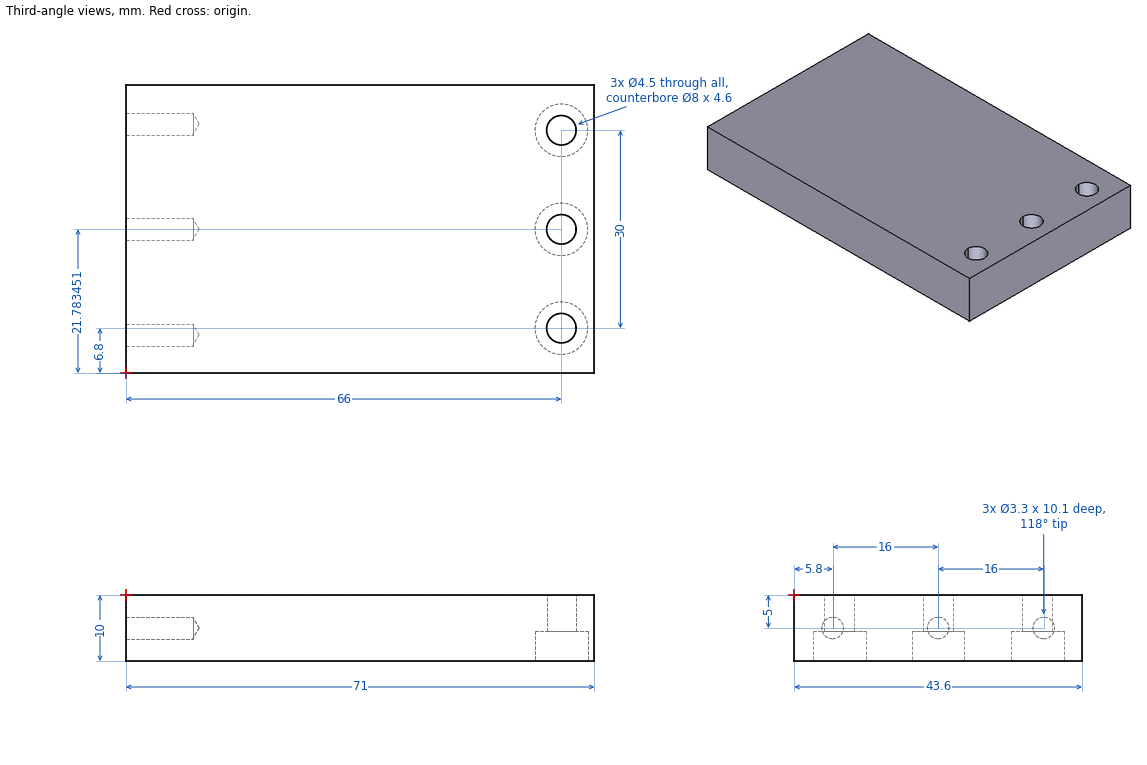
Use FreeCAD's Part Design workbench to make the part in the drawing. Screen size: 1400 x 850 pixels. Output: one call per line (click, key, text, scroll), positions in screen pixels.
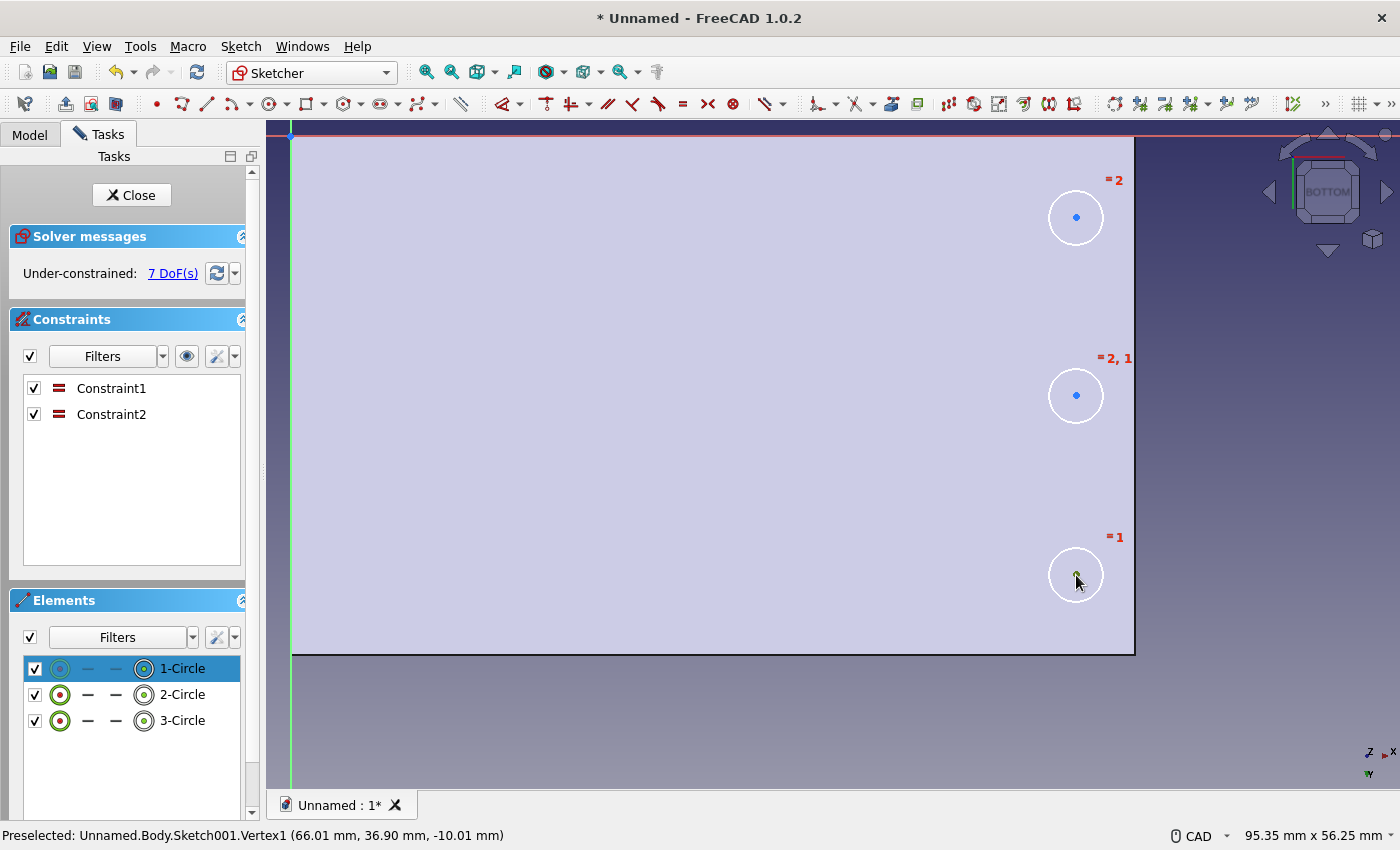
click(1076, 396)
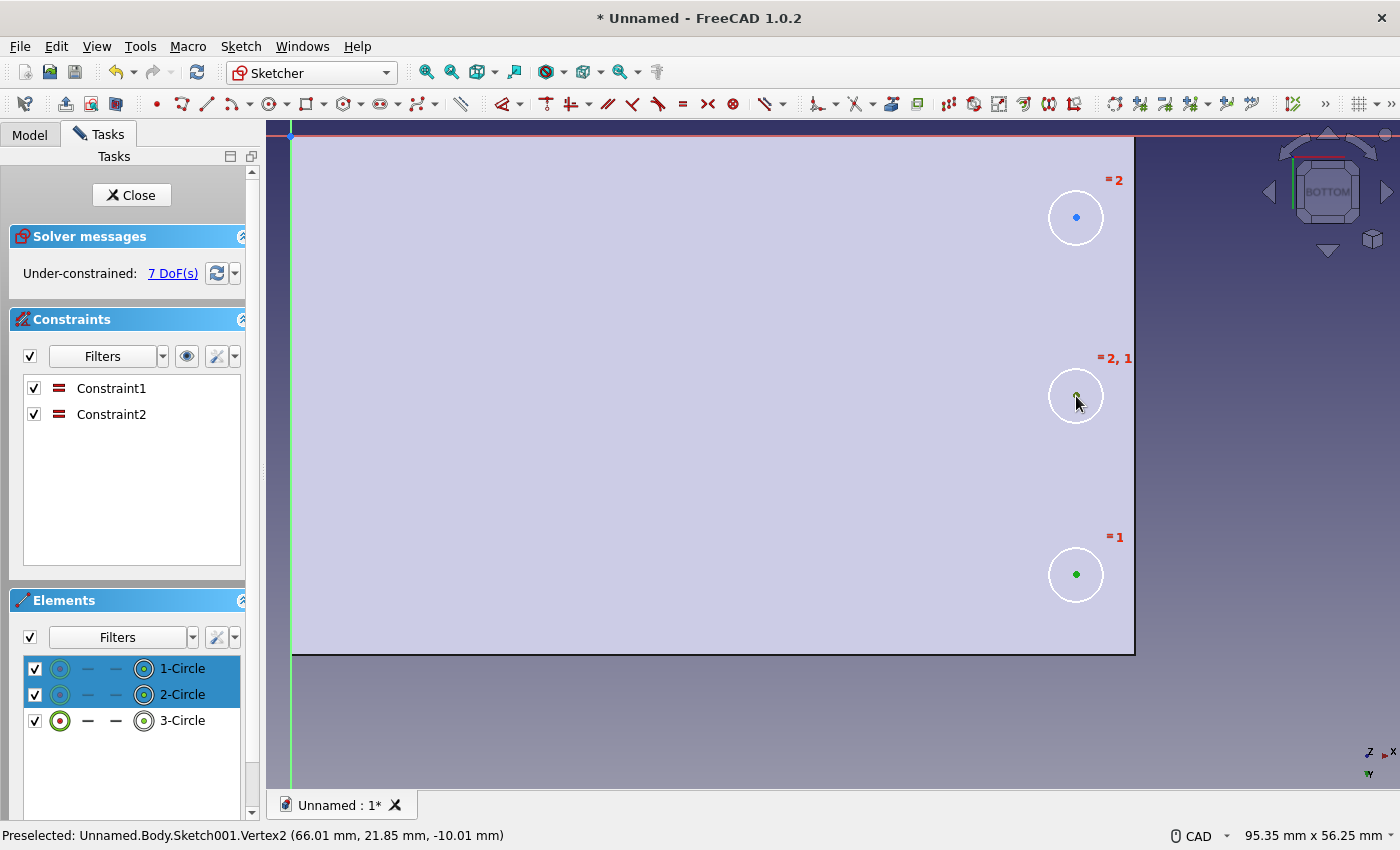
key(v)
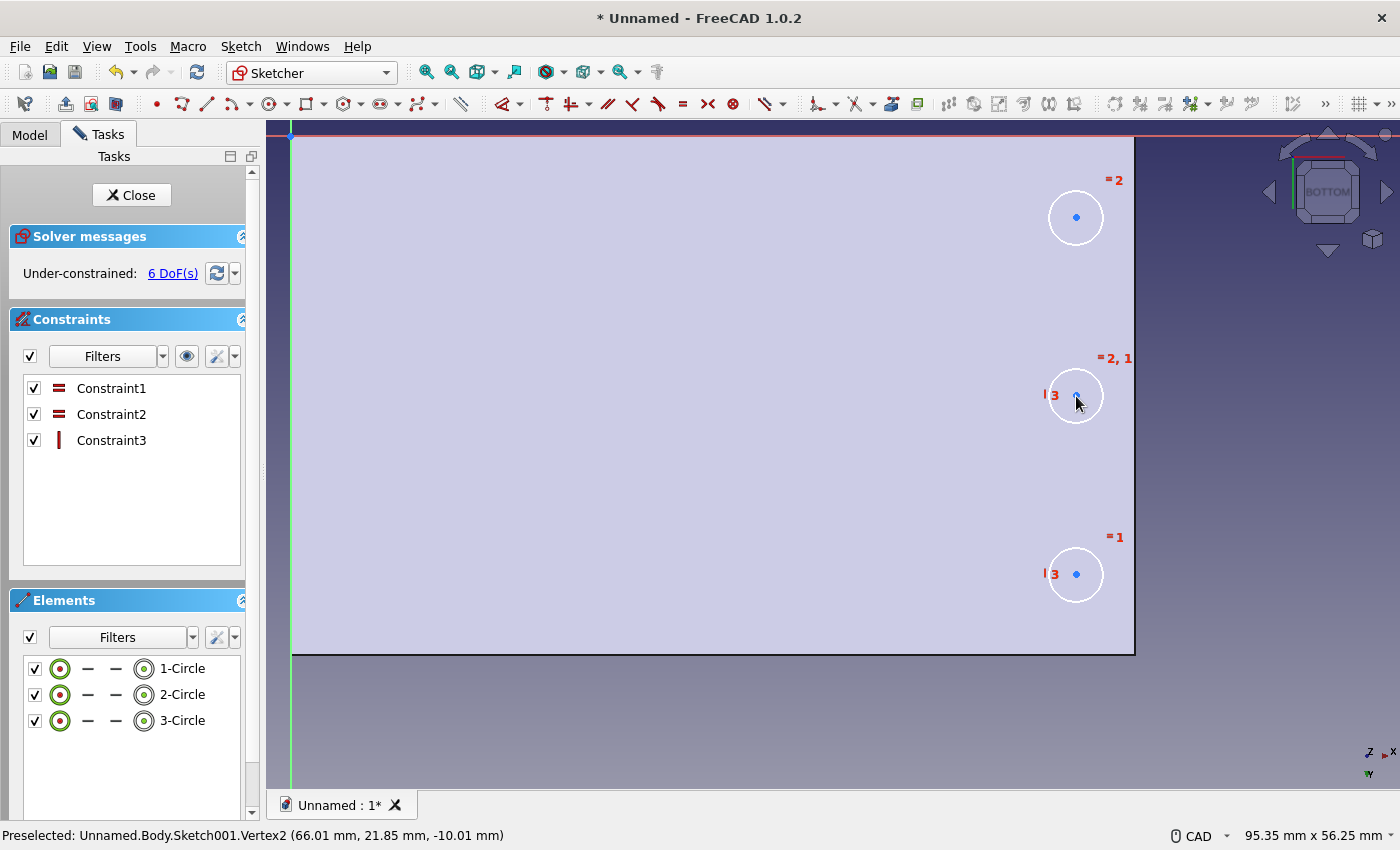
click(1076, 396)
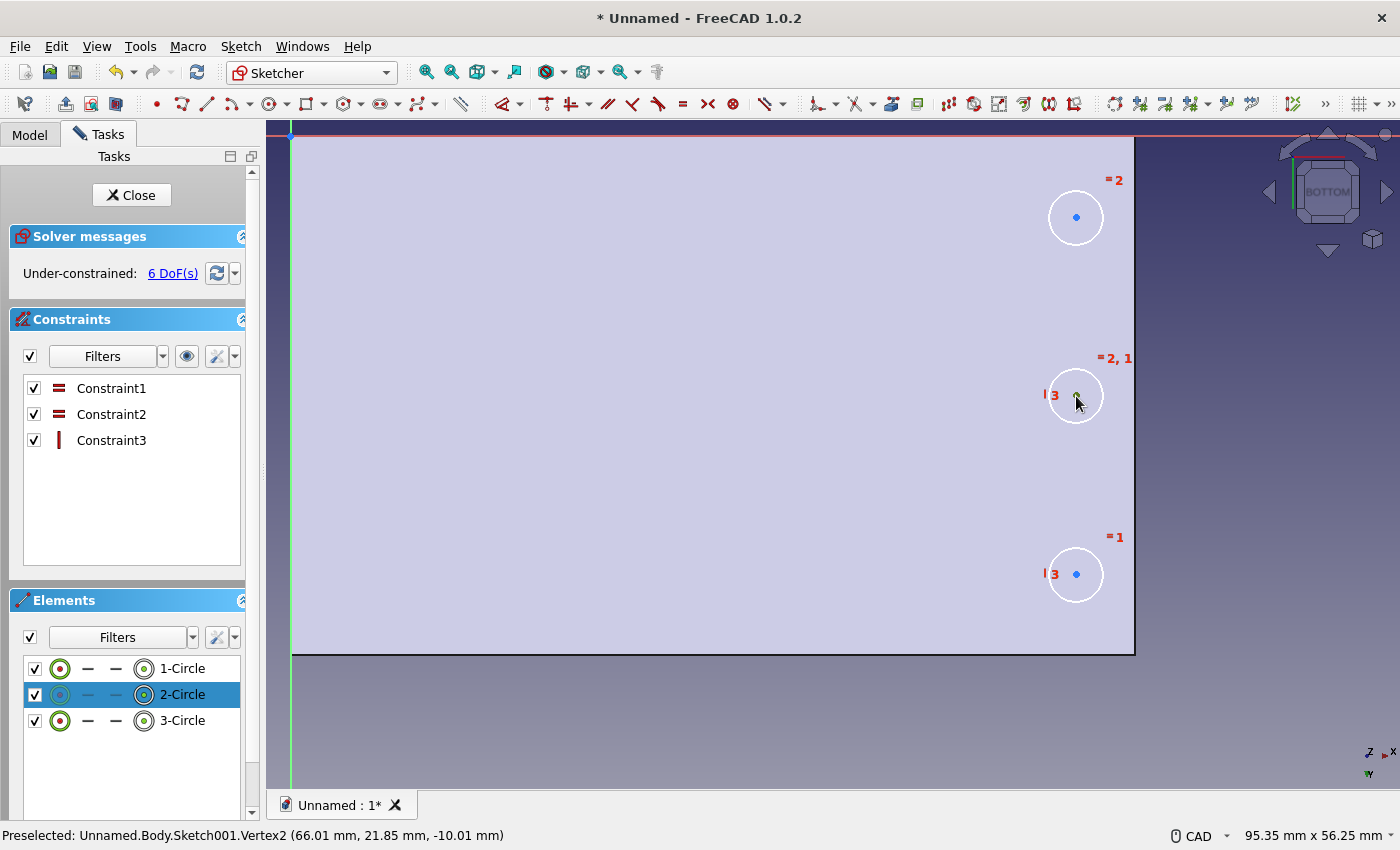
click(1076, 218)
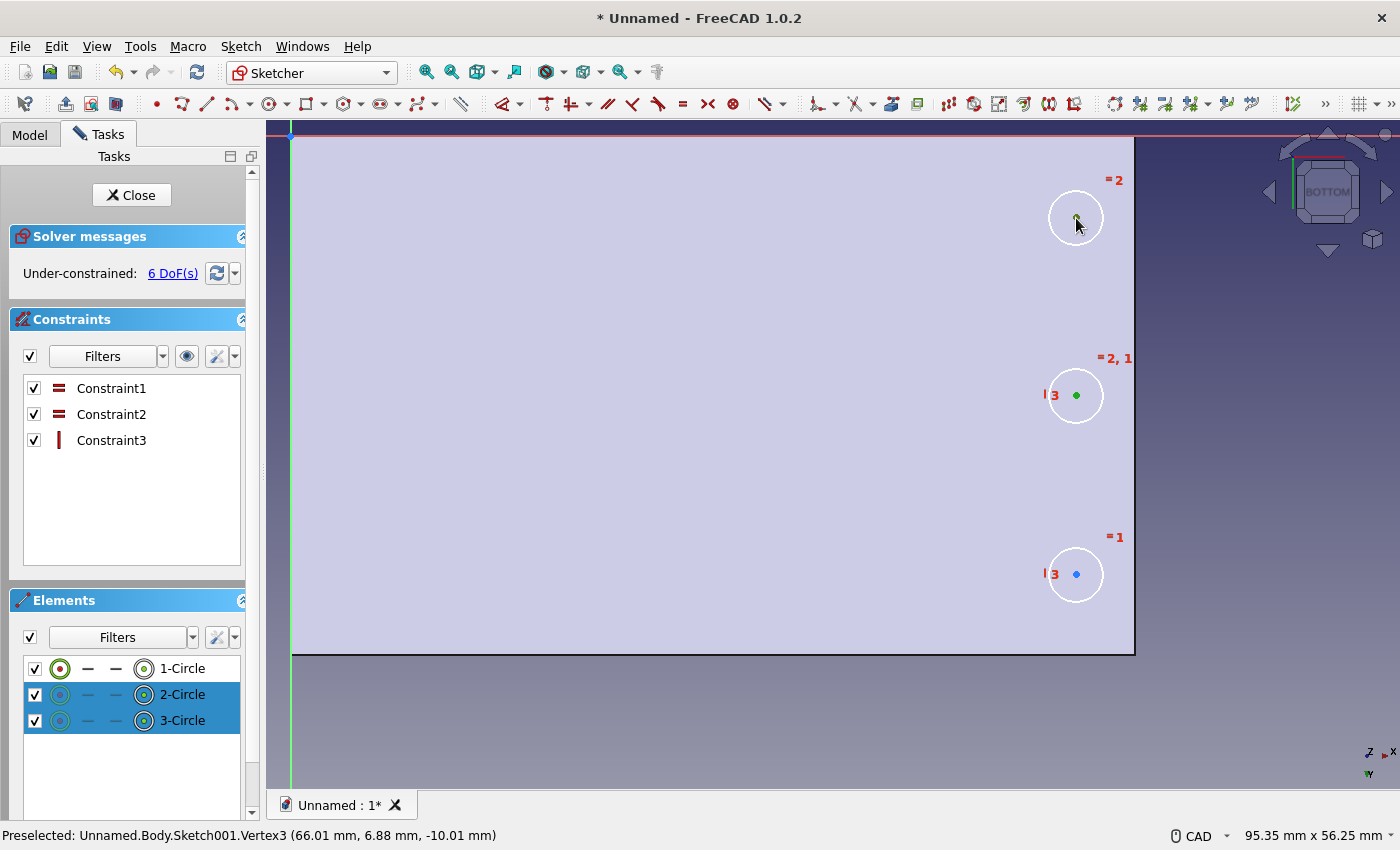
key(v)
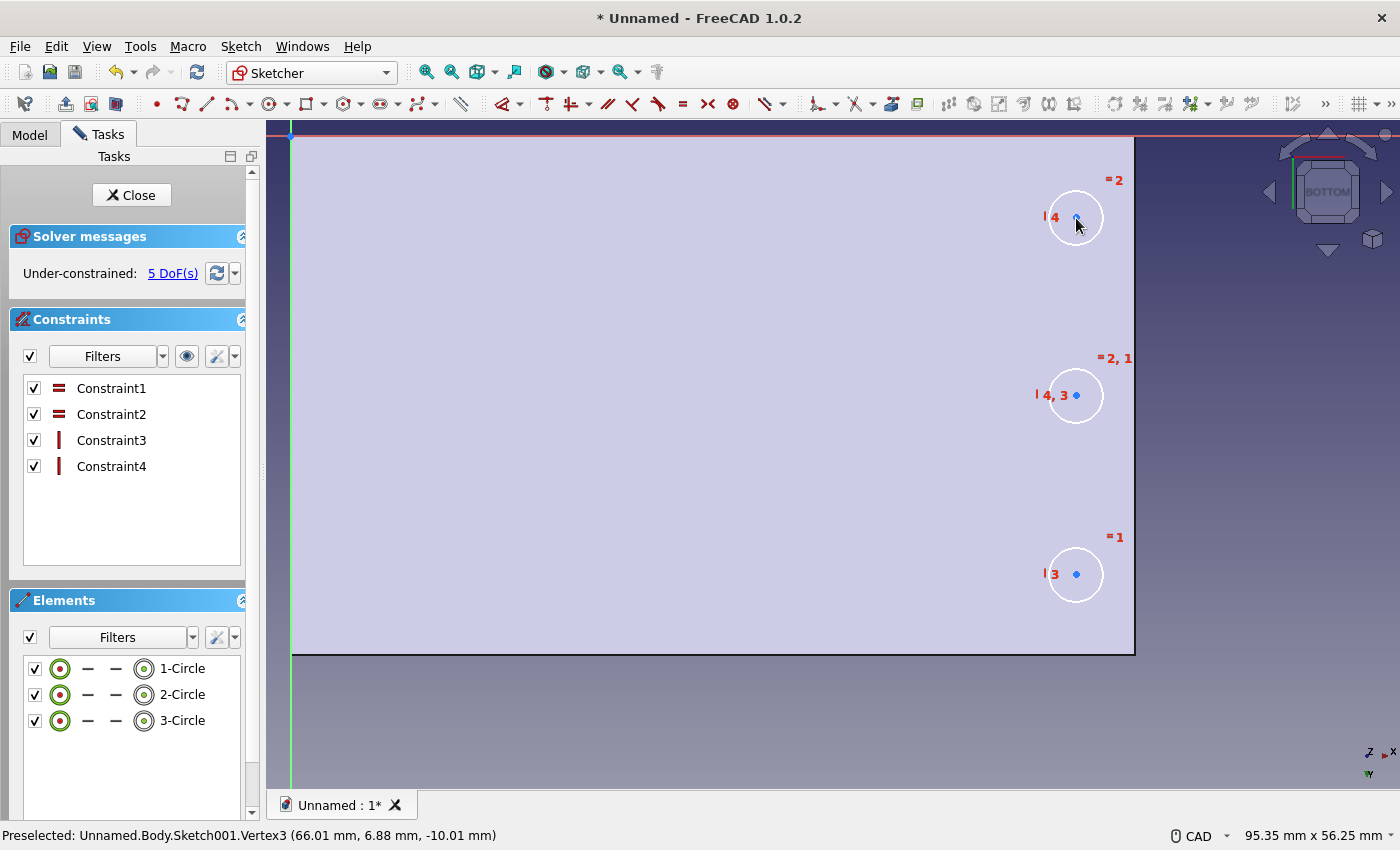
key(d)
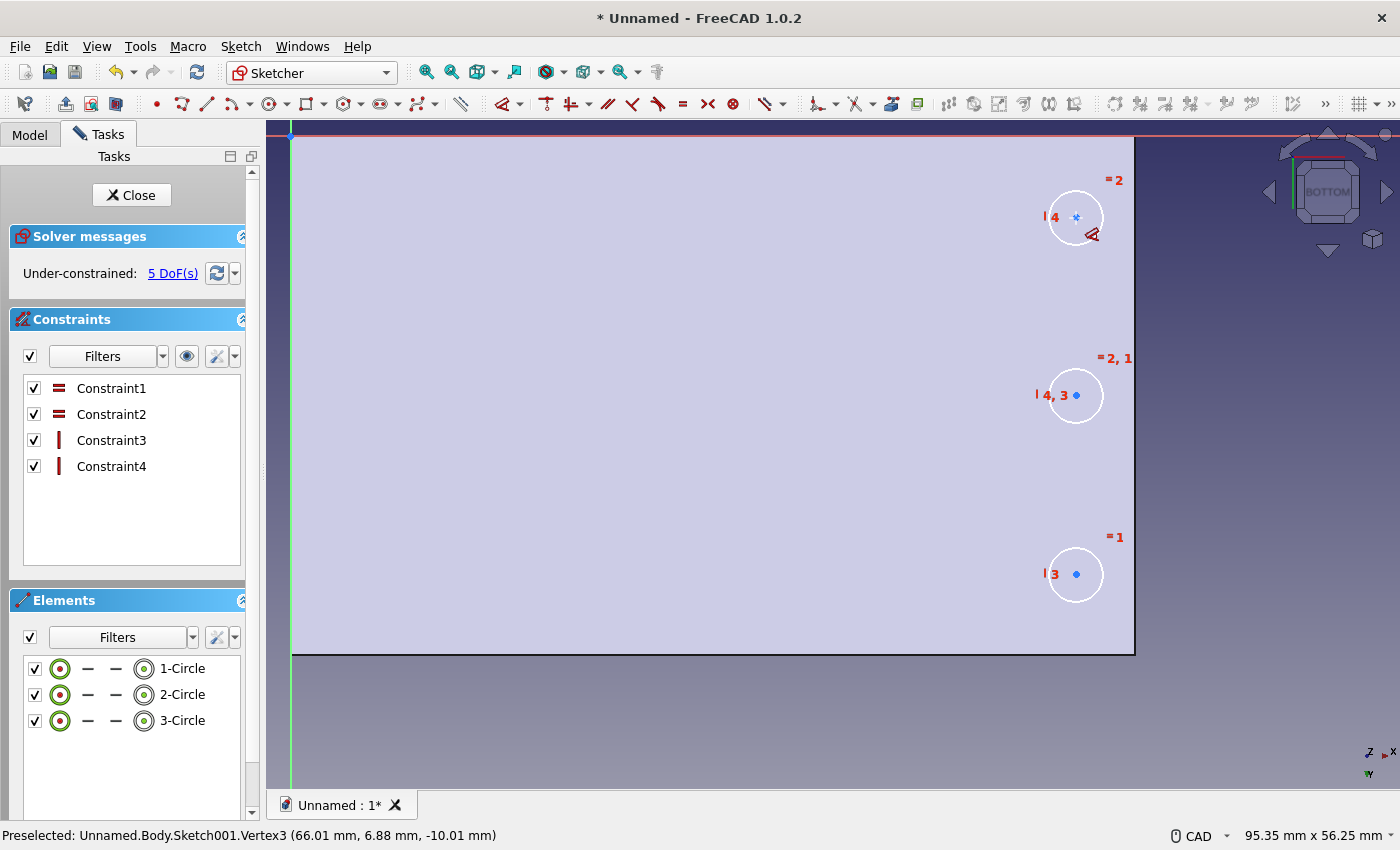
click(1095, 556)
click(1118, 533)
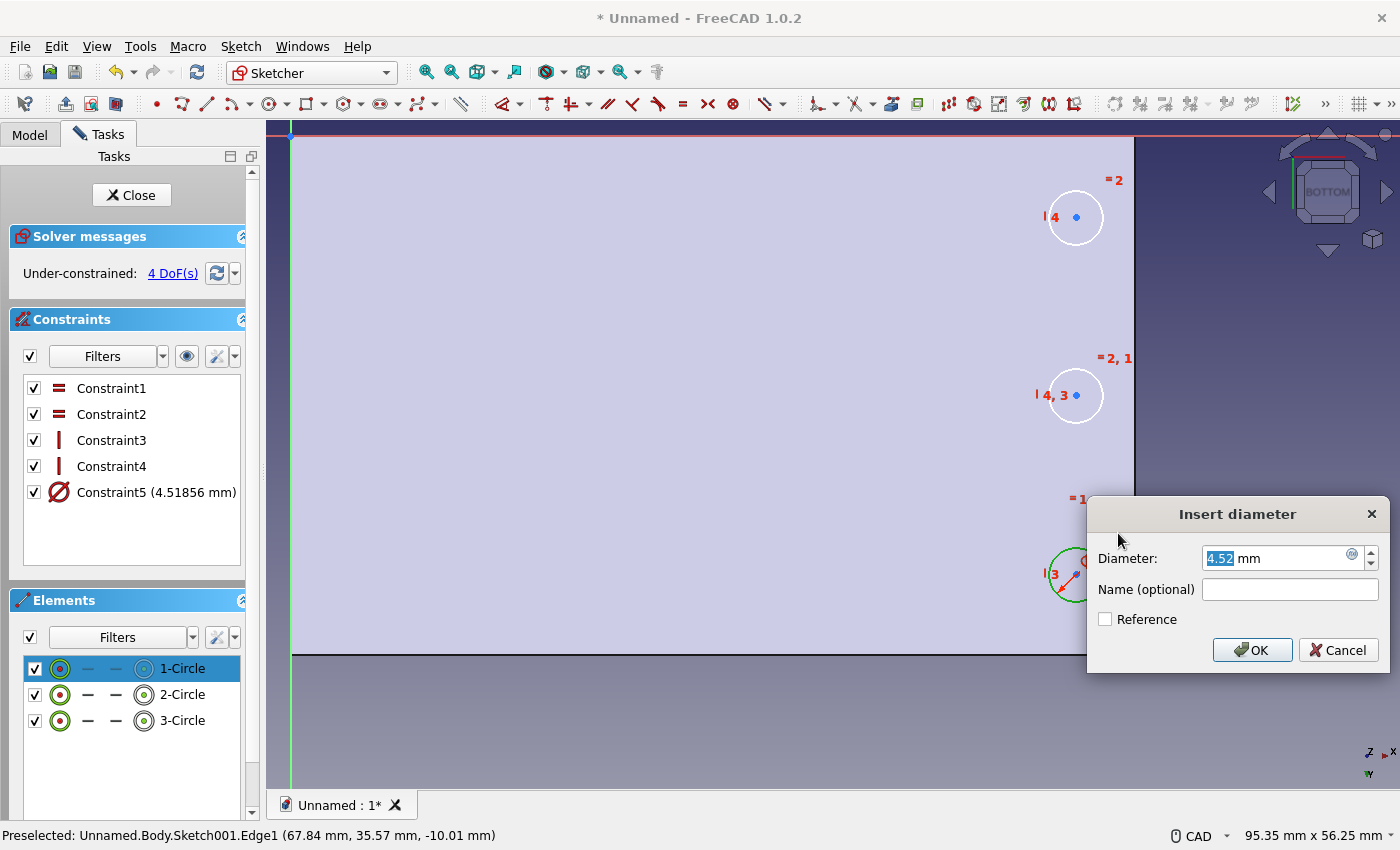
text(4.5)
key(Return)